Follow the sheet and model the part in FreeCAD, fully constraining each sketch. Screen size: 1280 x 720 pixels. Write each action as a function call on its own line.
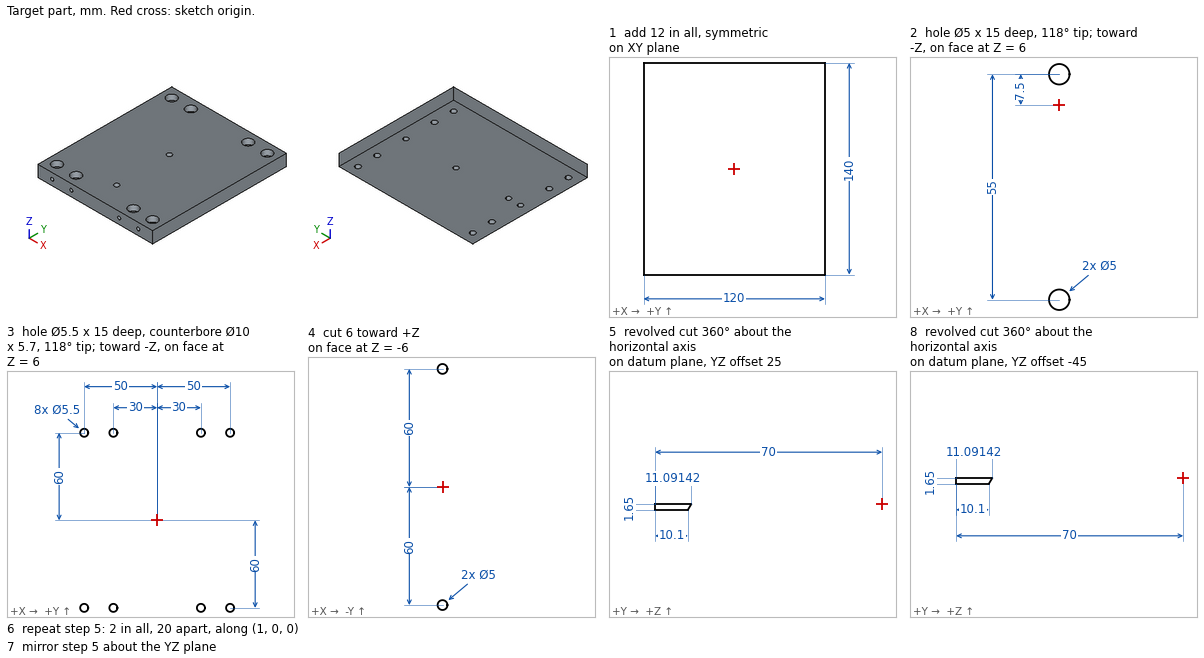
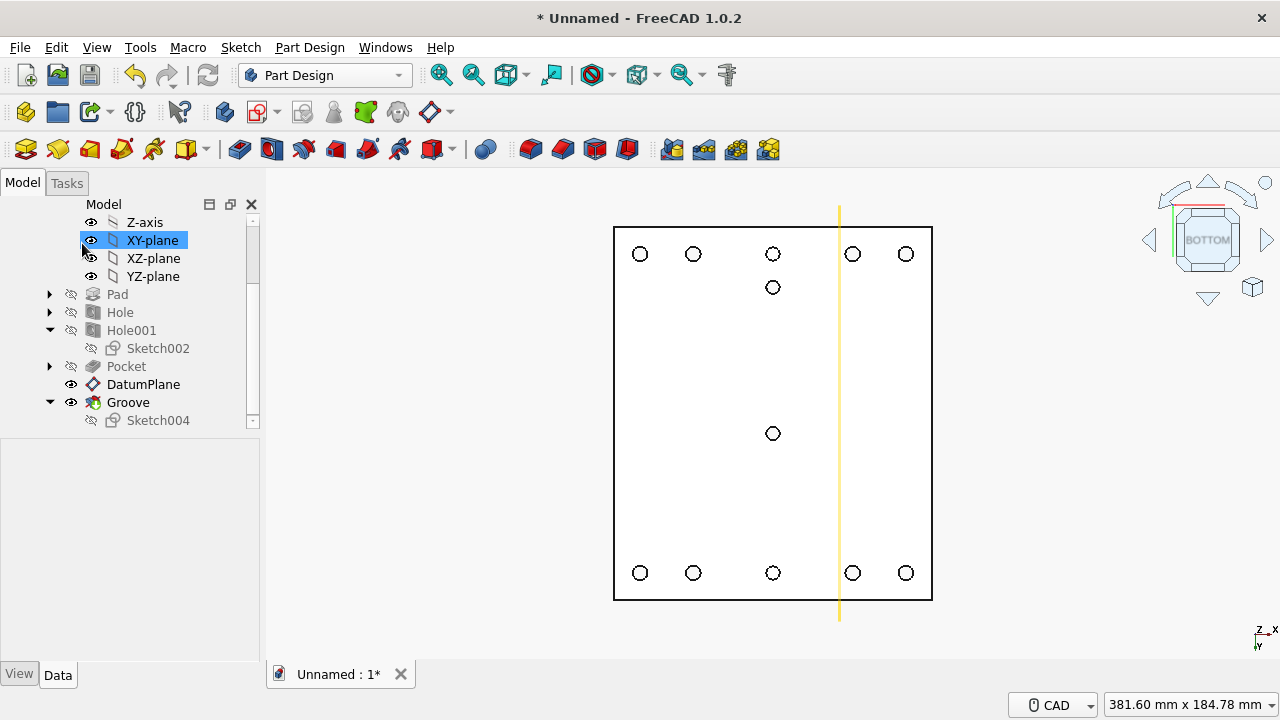
click(116, 384)
key(space)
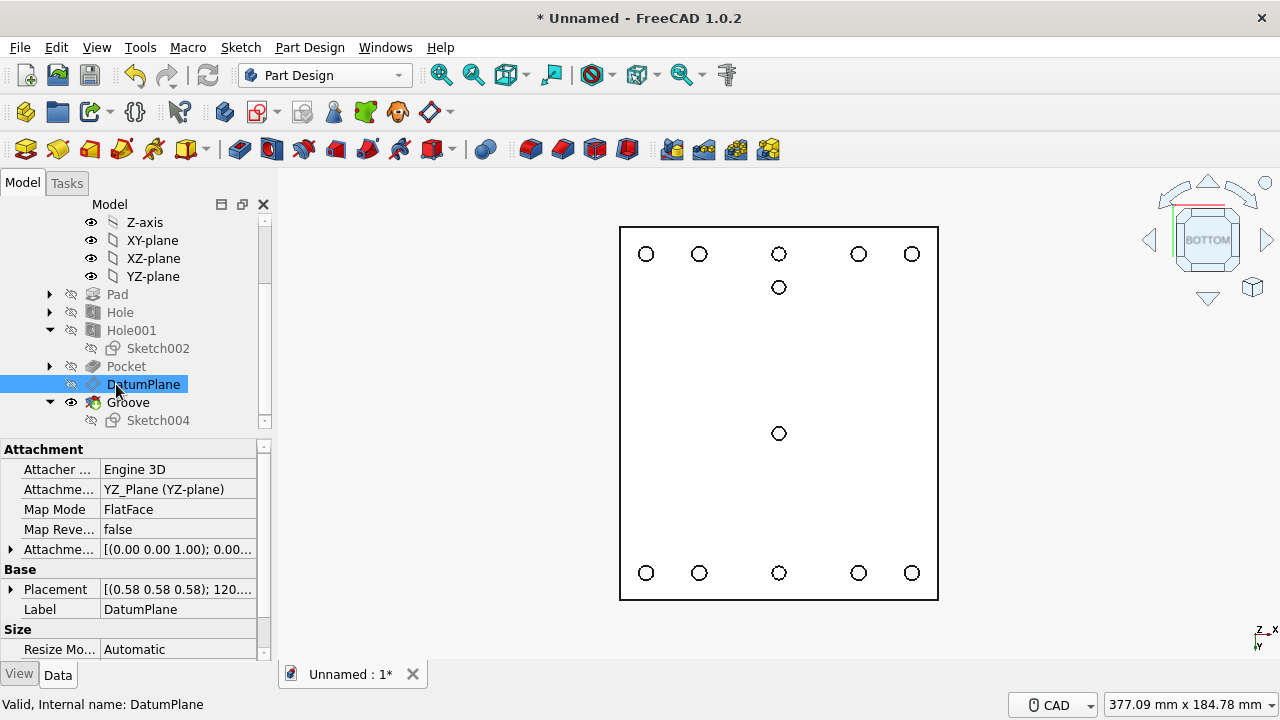
click(116, 402)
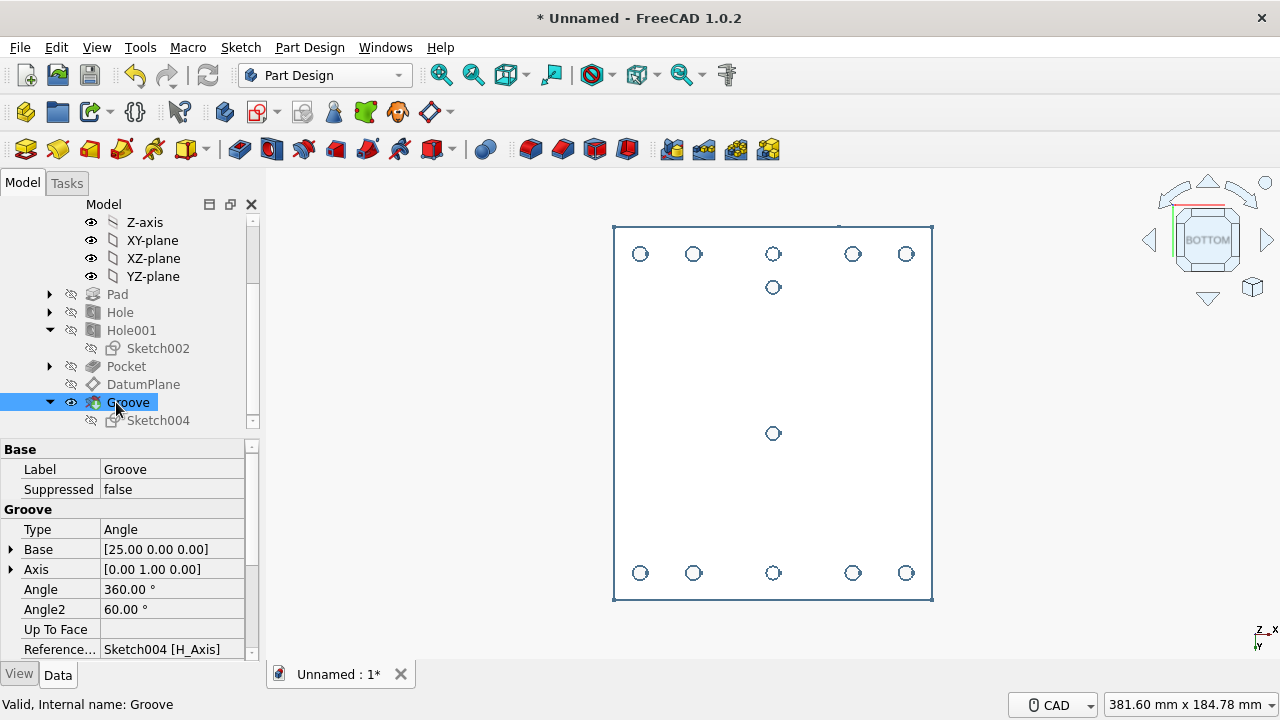
click(704, 150)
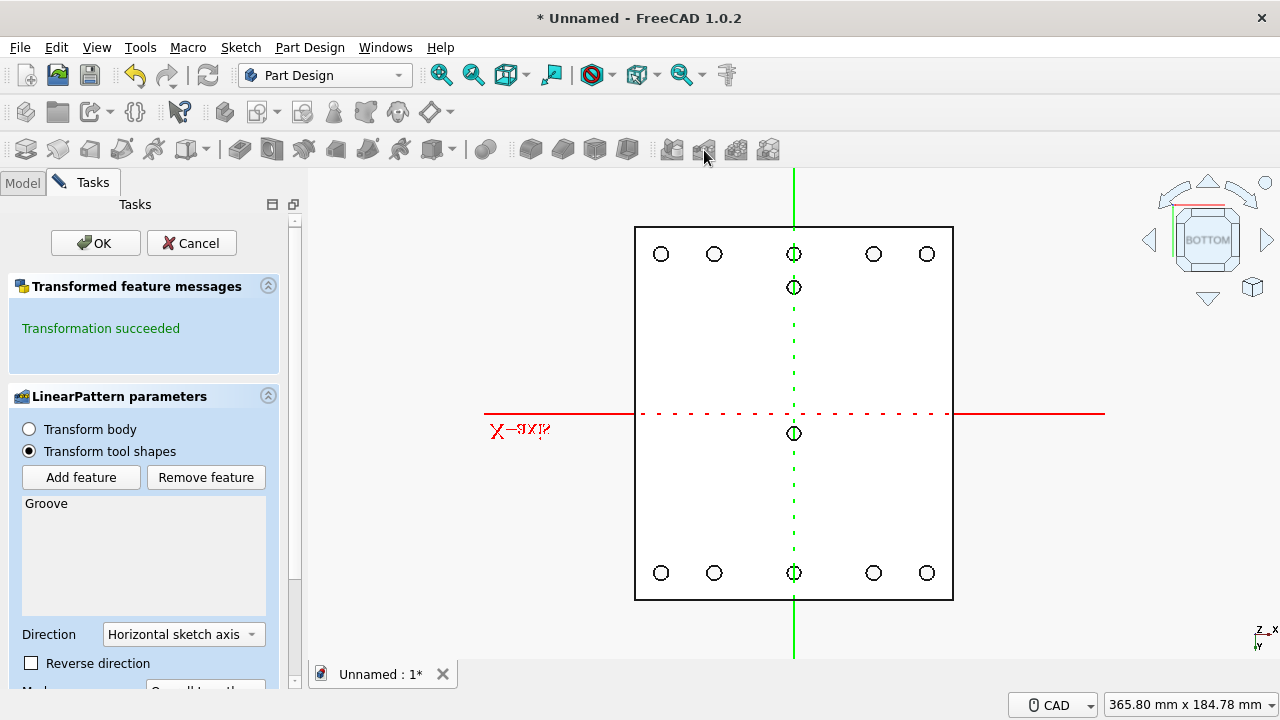
click(184, 634)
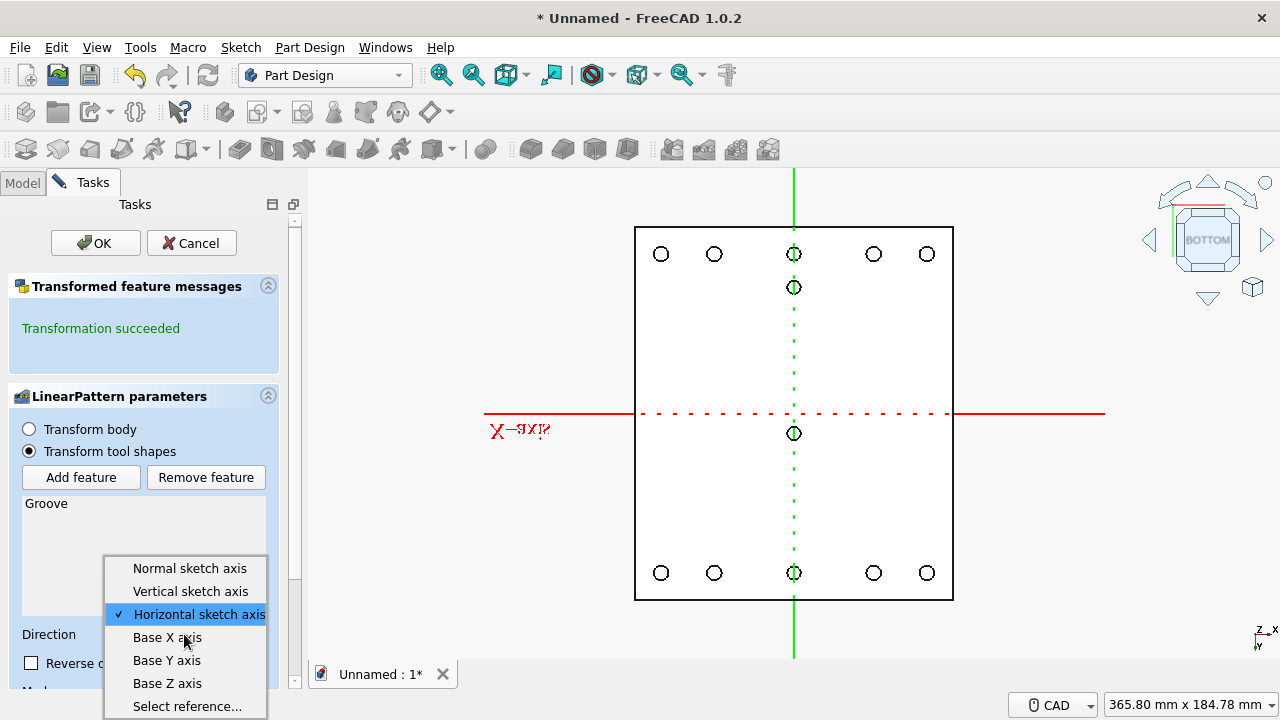
click(184, 638)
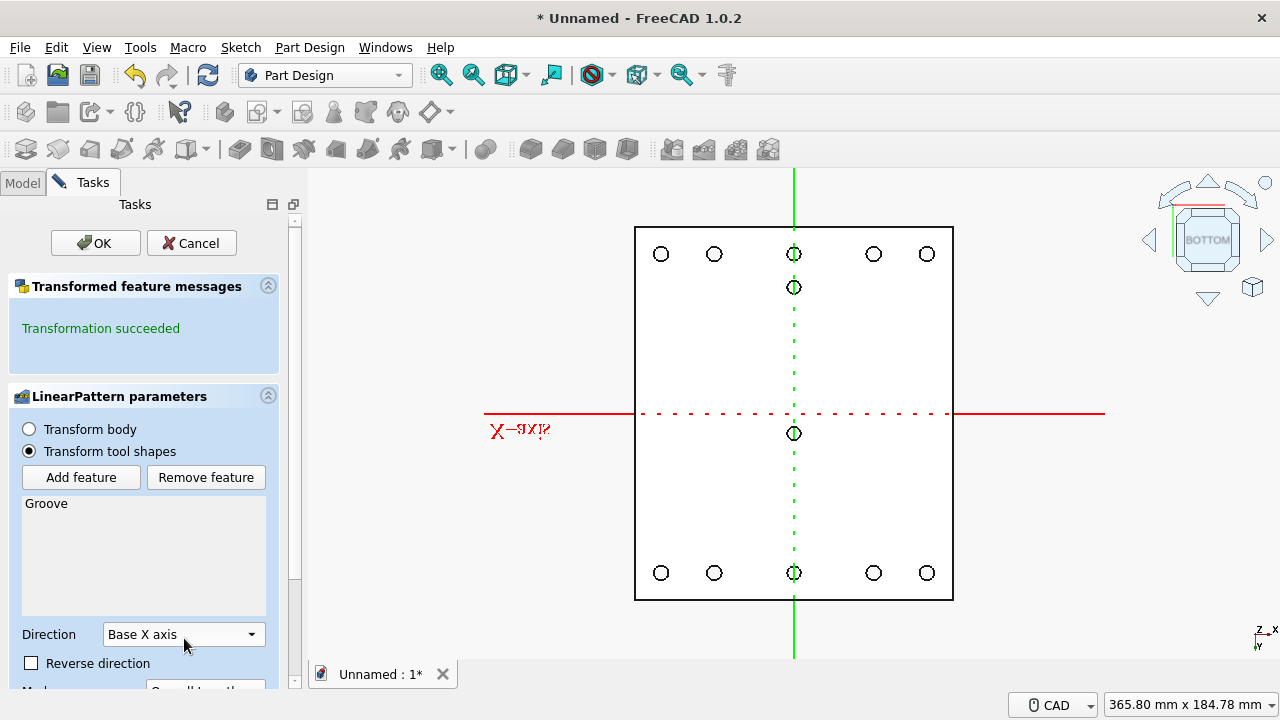
scroll(295, 451, down, 2)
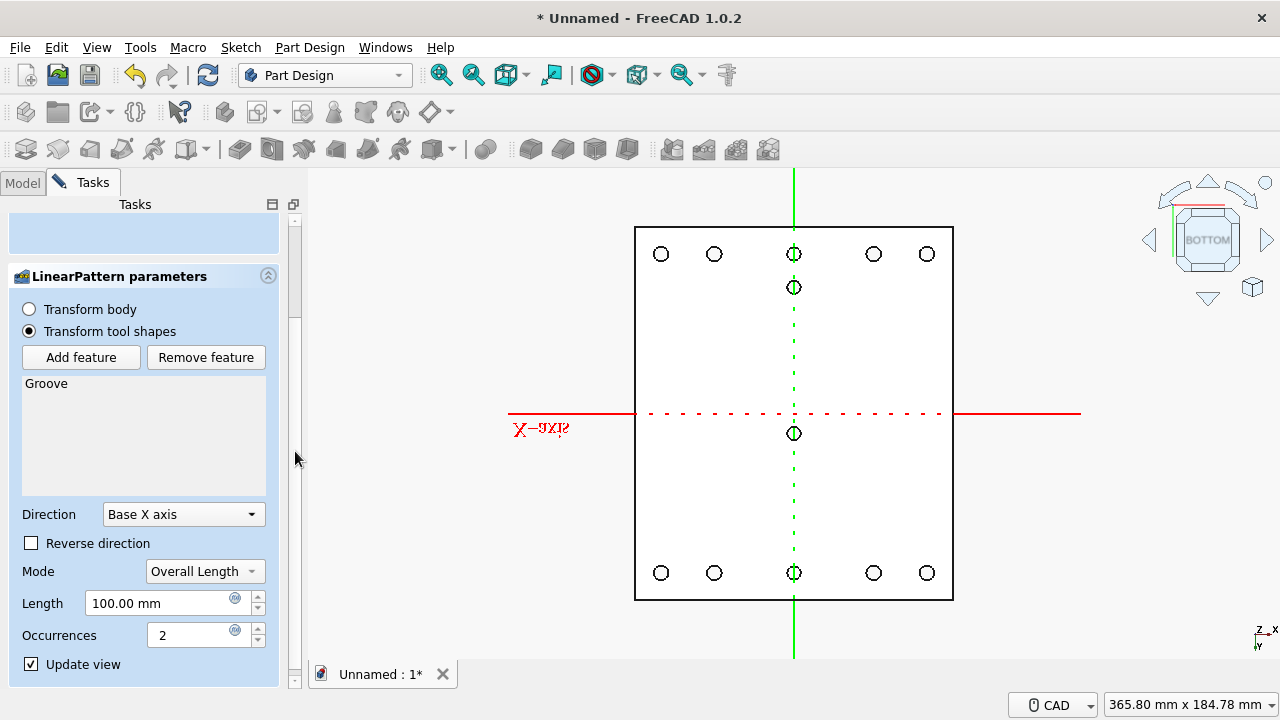
click(206, 572)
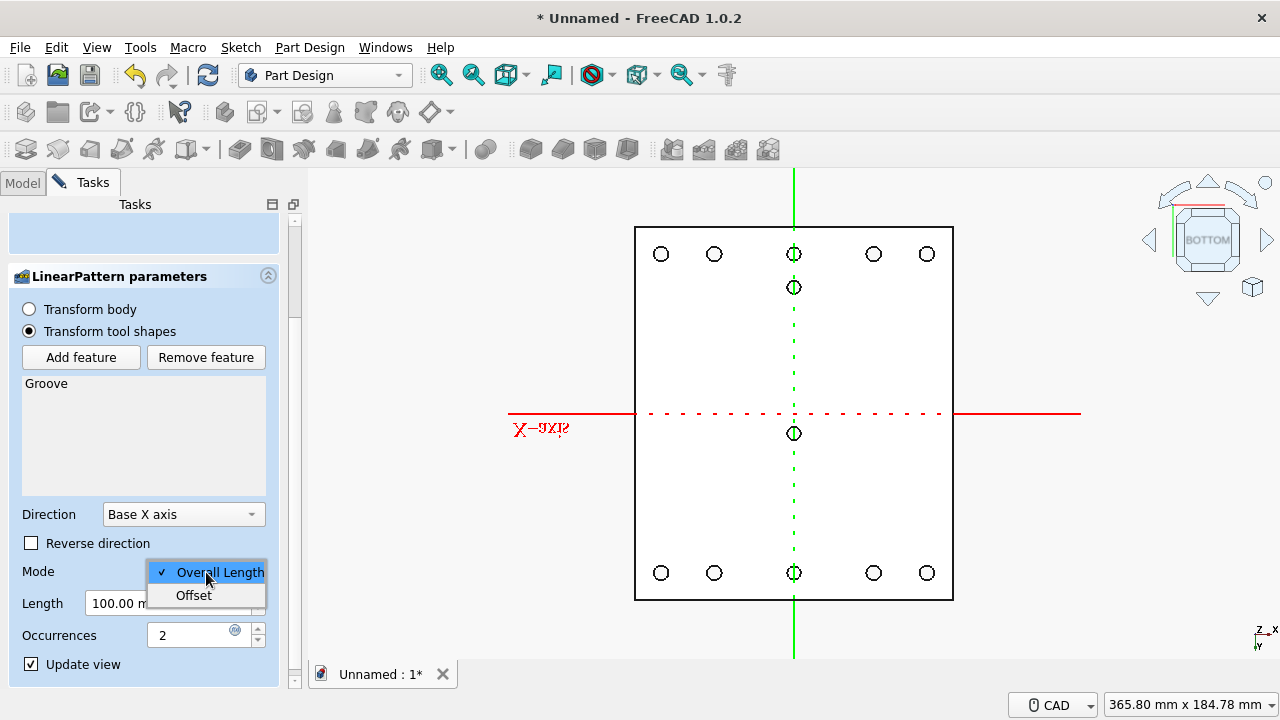
click(206, 596)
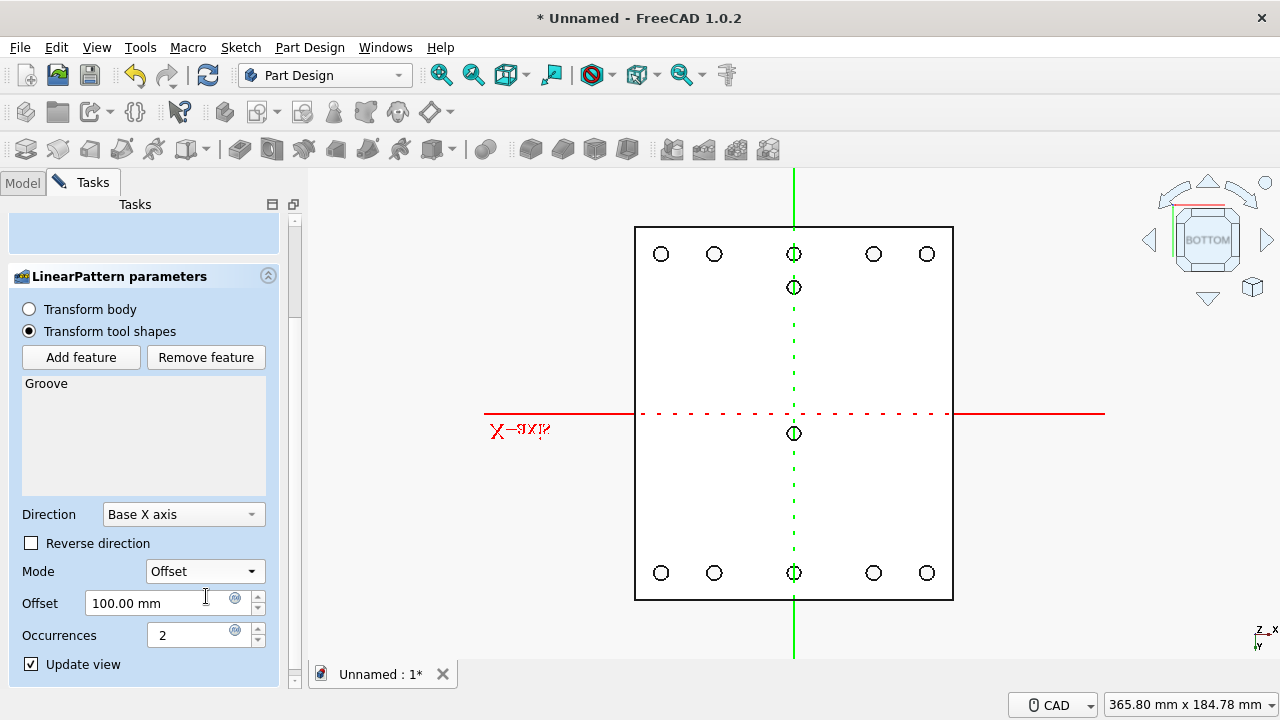
triple_click(168, 603)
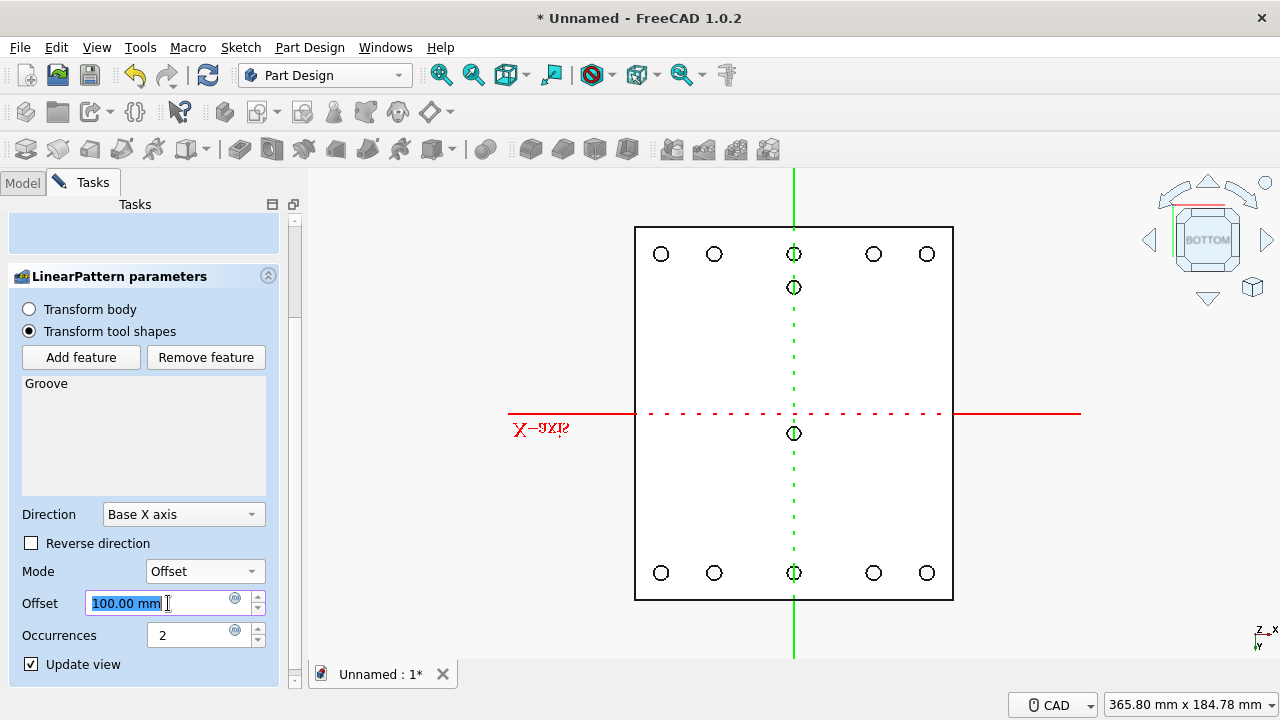
text(20)
key(Tab)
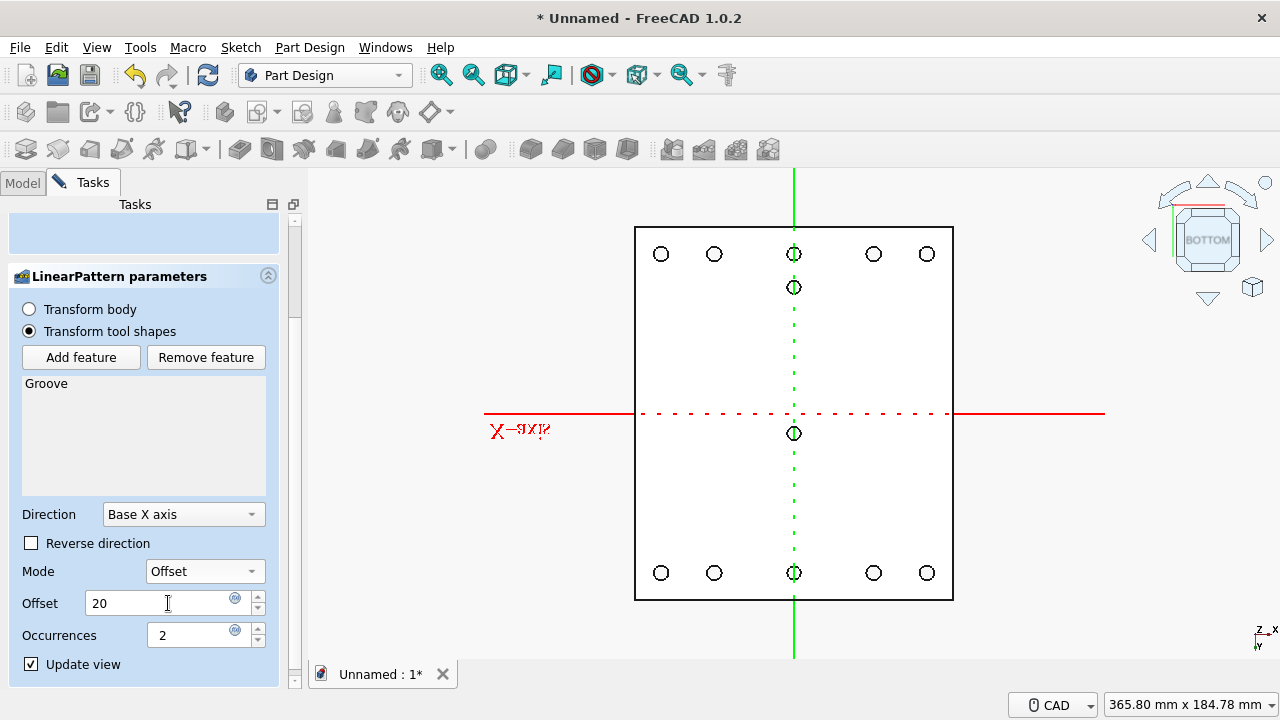
triple_click(198, 635)